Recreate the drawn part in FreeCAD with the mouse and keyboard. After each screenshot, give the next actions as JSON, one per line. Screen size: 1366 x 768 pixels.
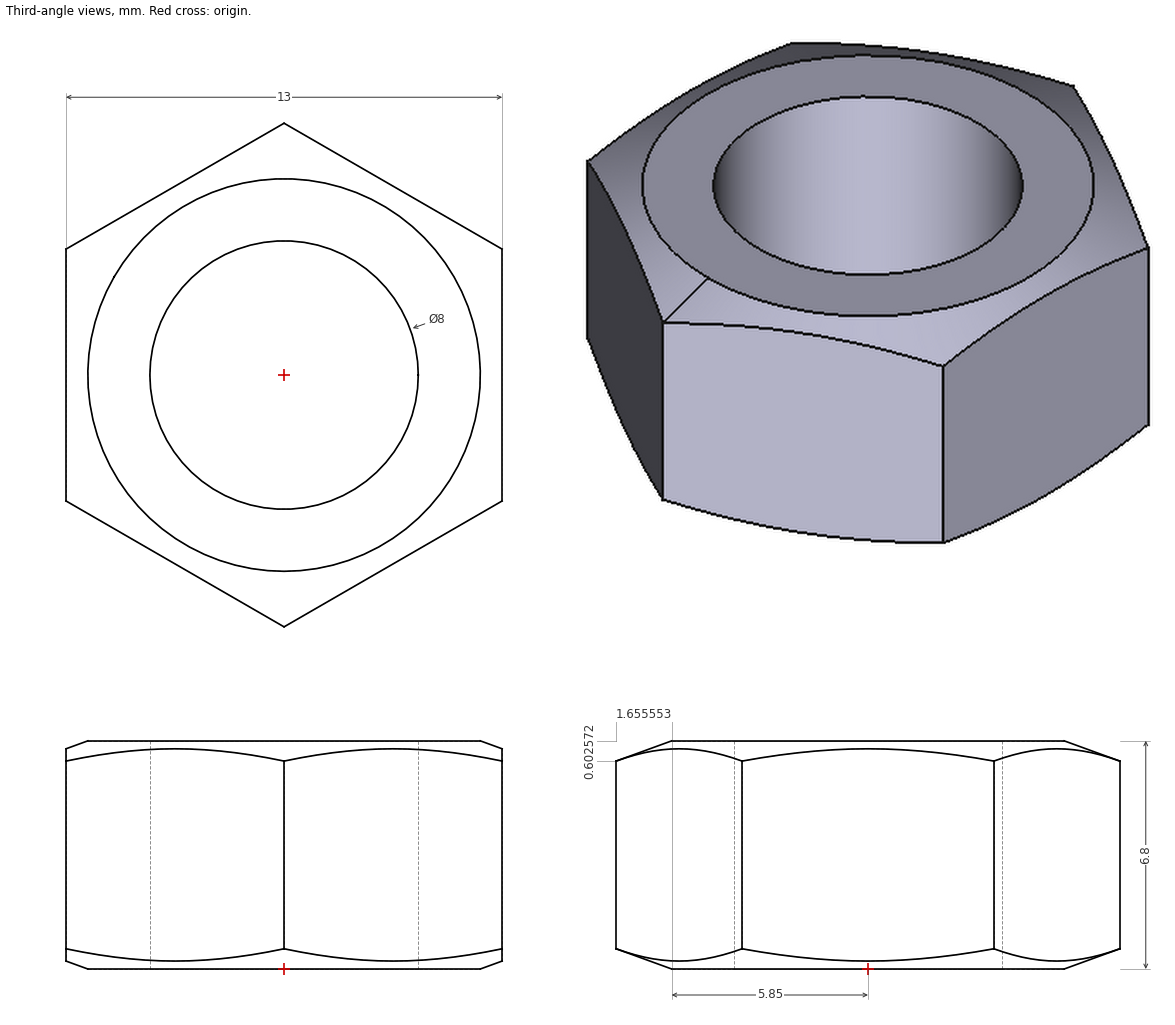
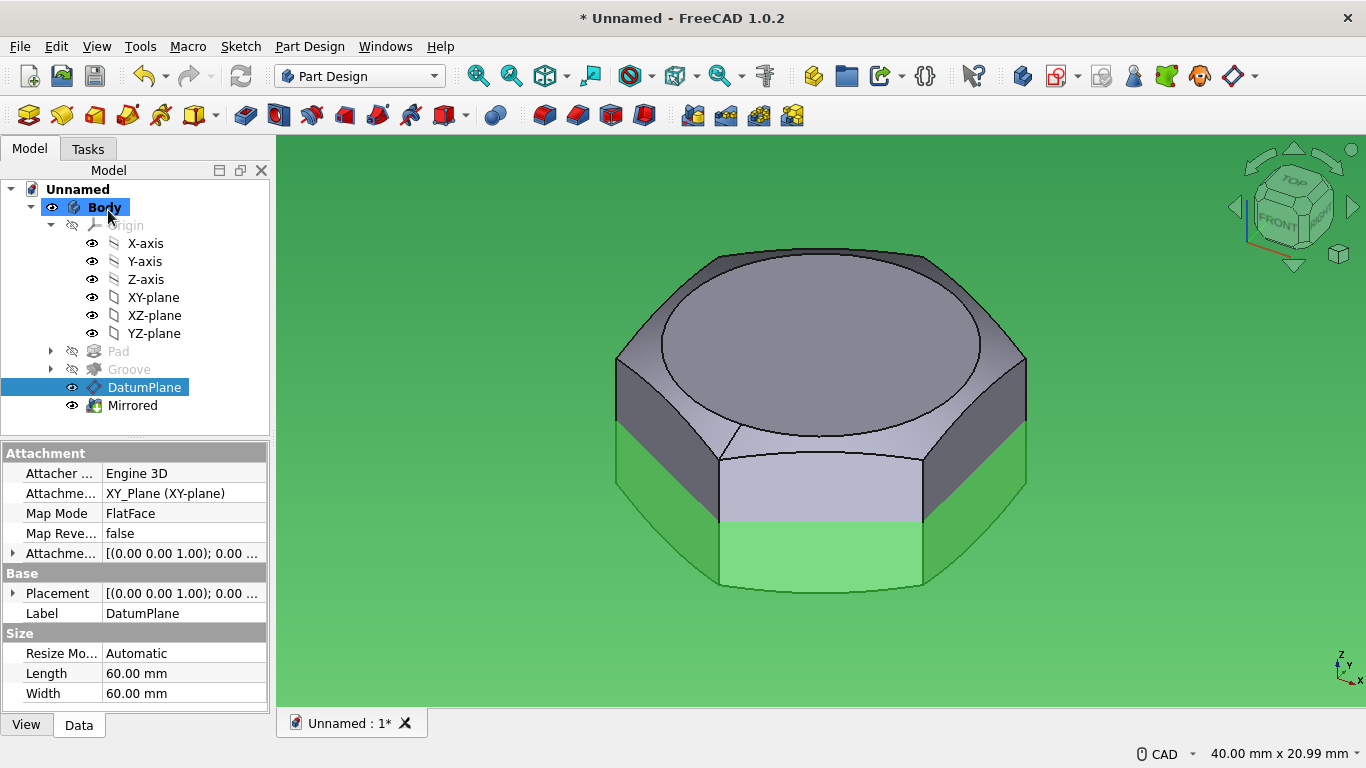
{"action": "left_click", "coordinate": [117, 387]}
{"action": "key", "text": "space"}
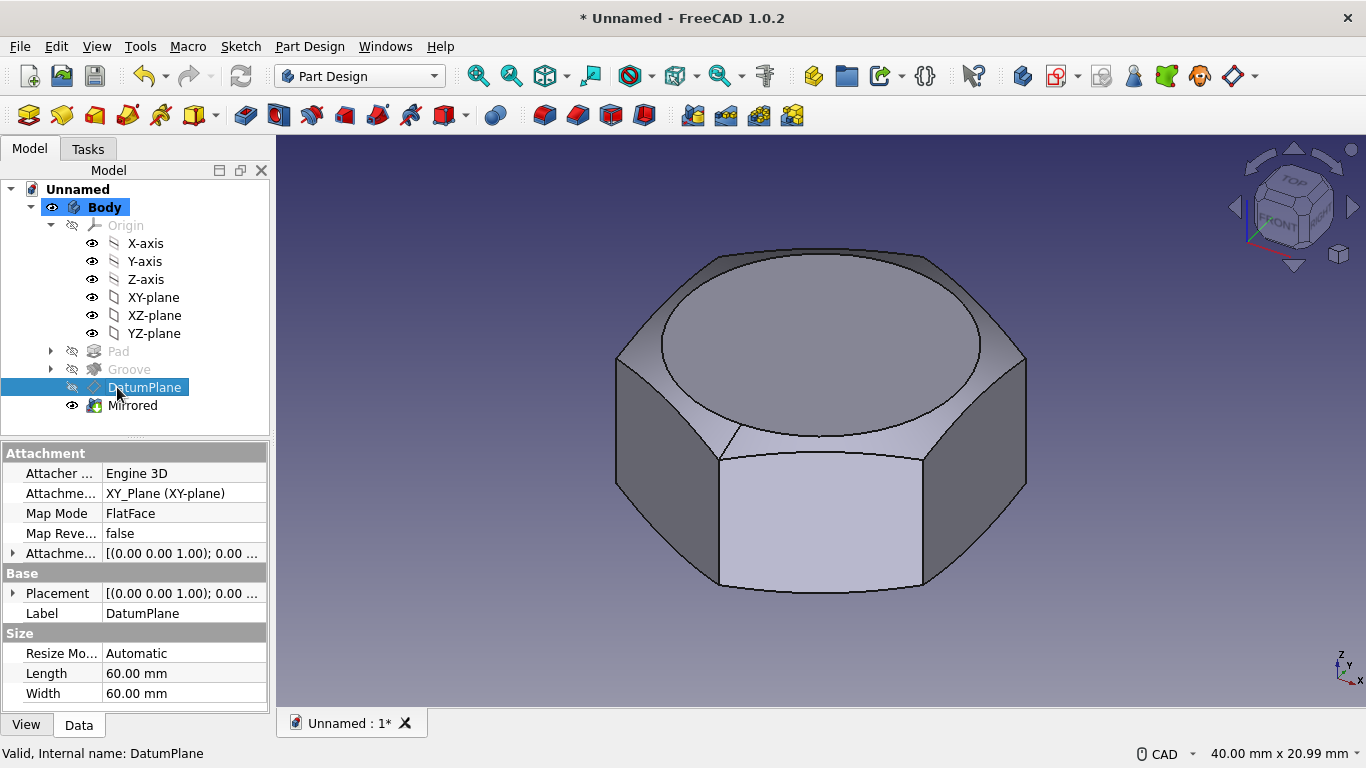
{"action": "left_click", "coordinate": [821, 344]}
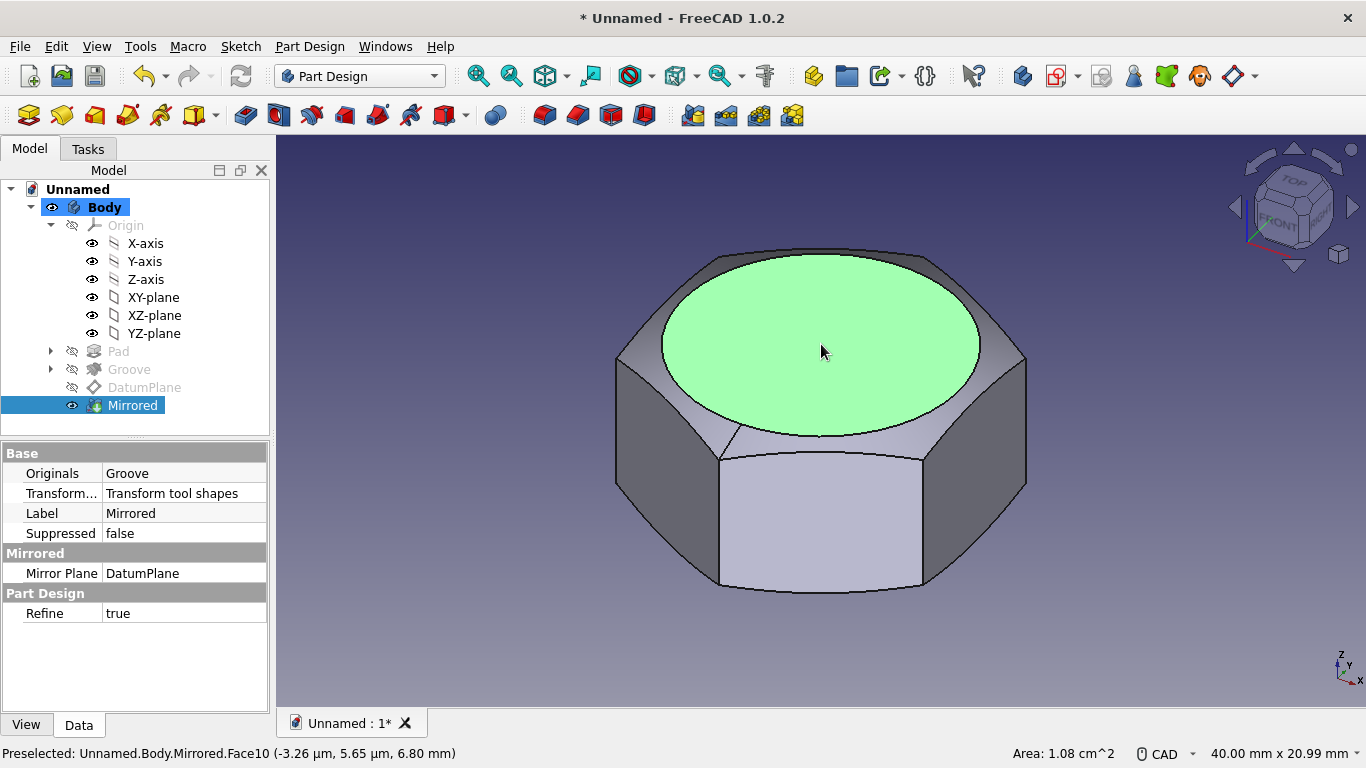
{"action": "left_click", "coordinate": [1056, 76]}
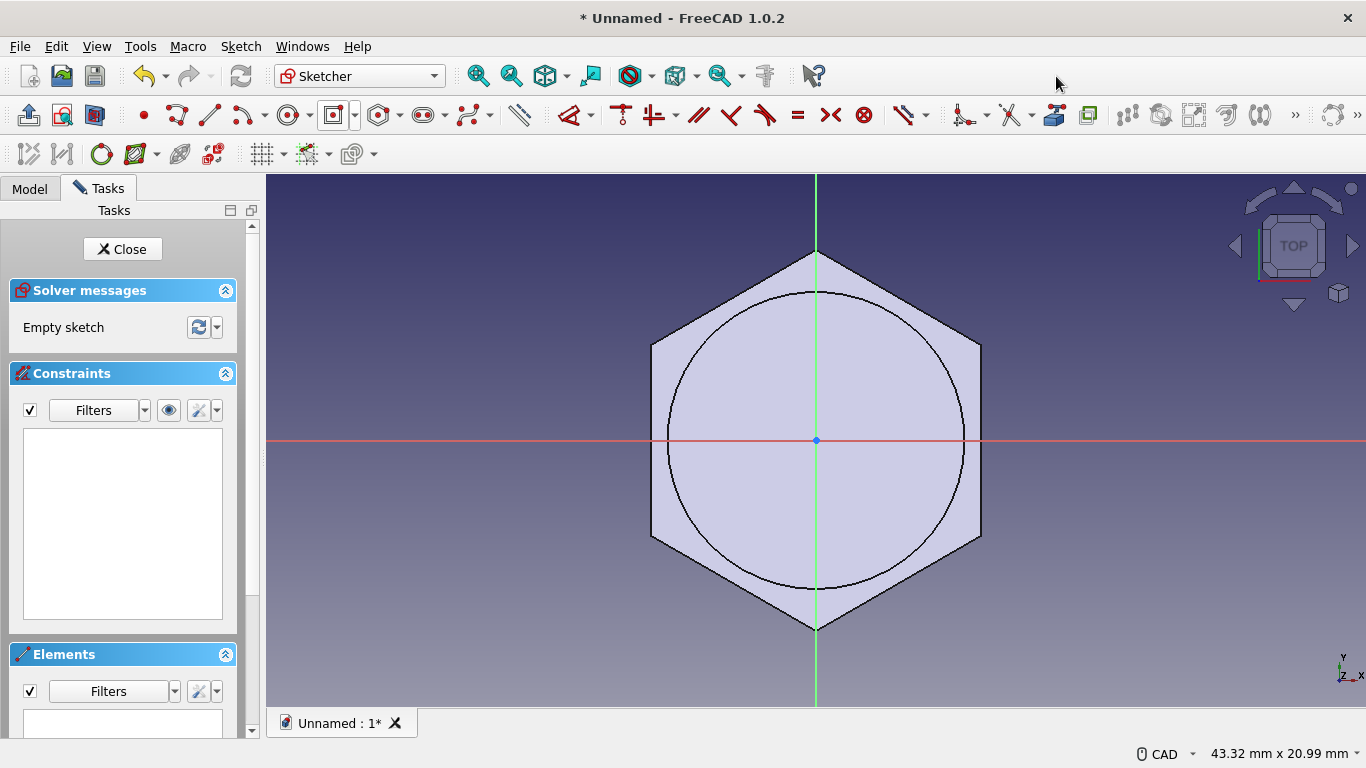
{"action": "scroll", "coordinate": [899, 441], "scroll_direction": "up", "scroll_amount": 3}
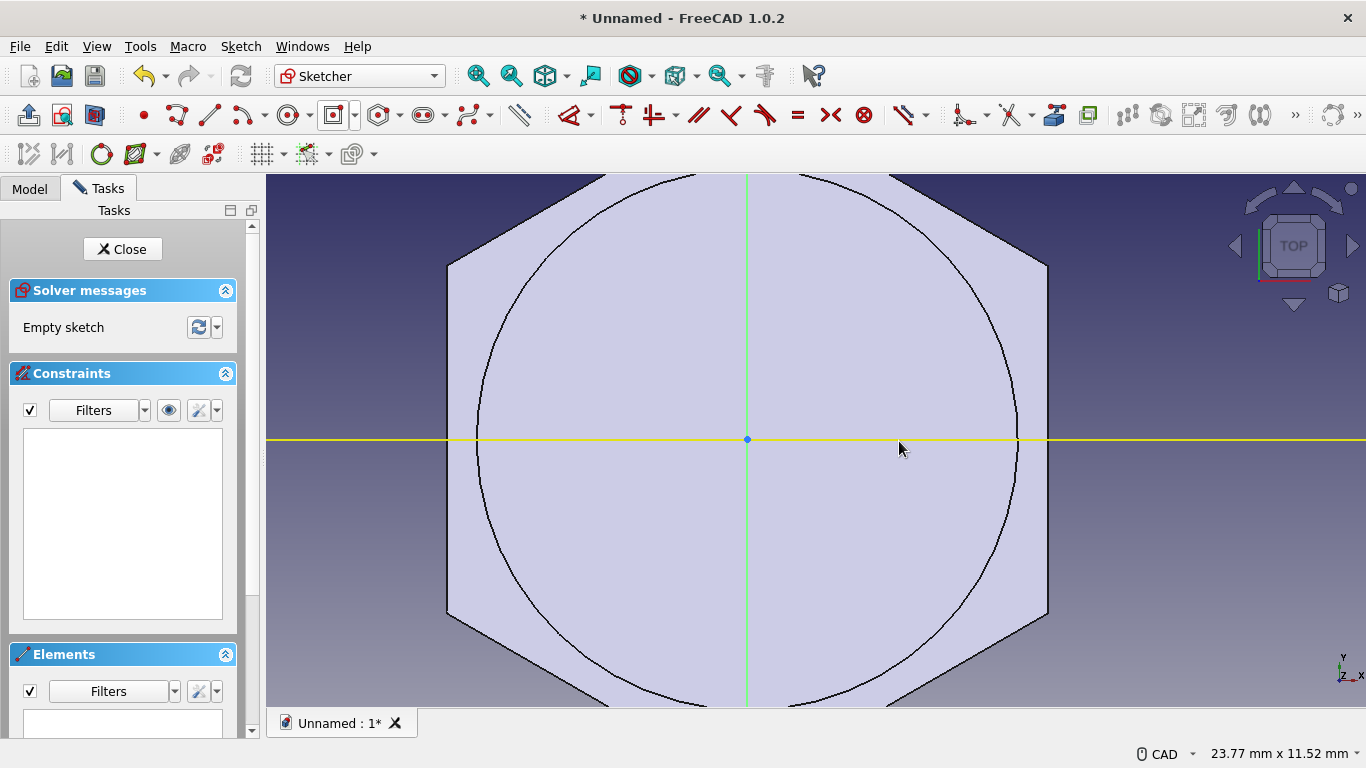
{"action": "left_click", "coordinate": [288, 116]}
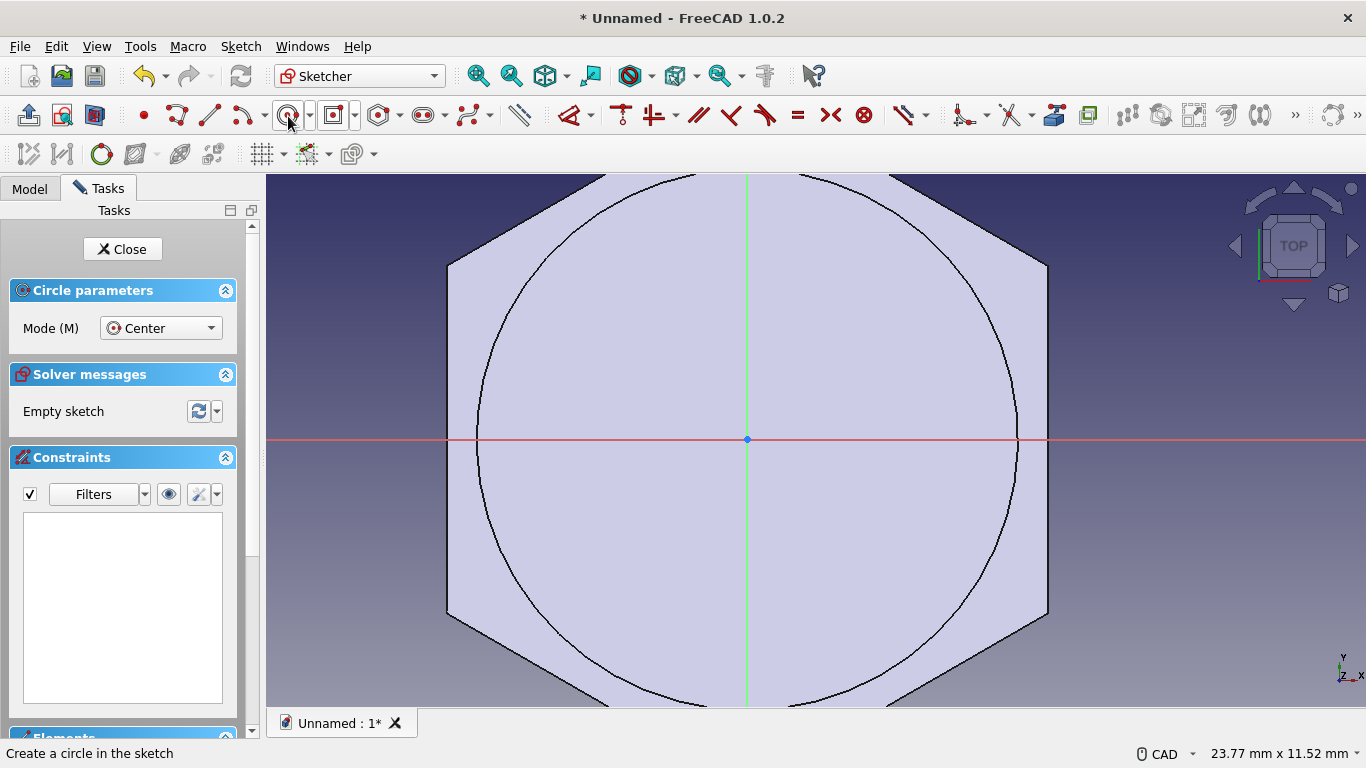
{"action": "left_click", "coordinate": [747, 440]}
{"action": "left_click", "coordinate": [878, 309]}
{"action": "key", "text": "Escape"}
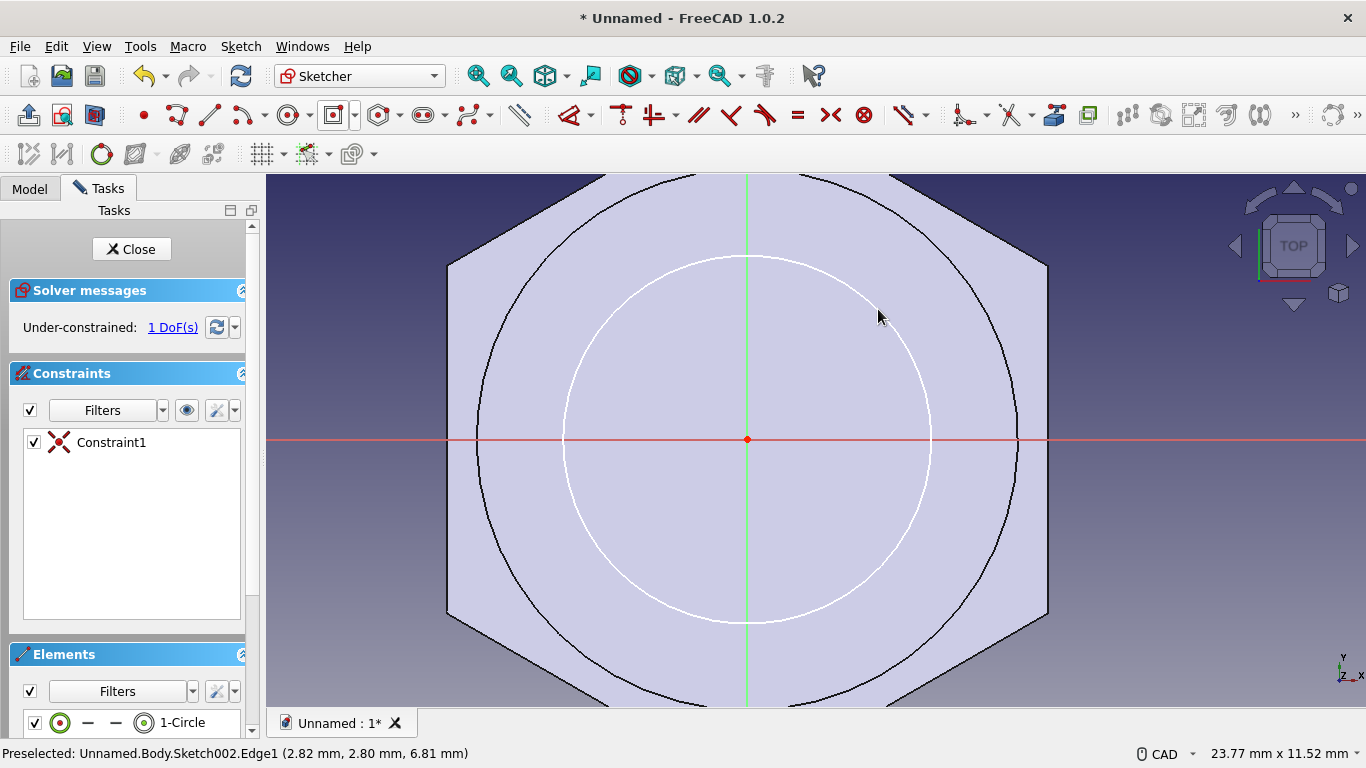
{"action": "key", "text": "d"}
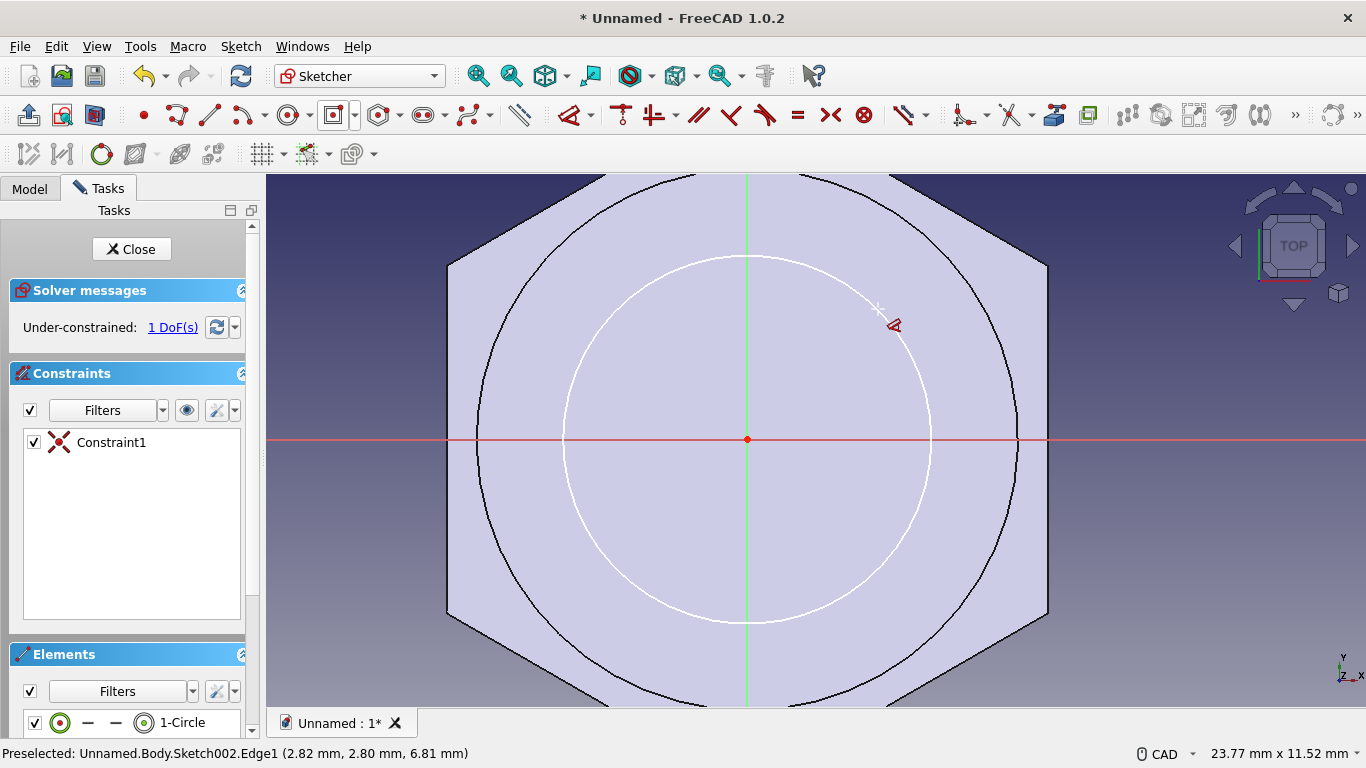
{"action": "left_click", "coordinate": [877, 309]}
{"action": "left_click", "coordinate": [900, 286]}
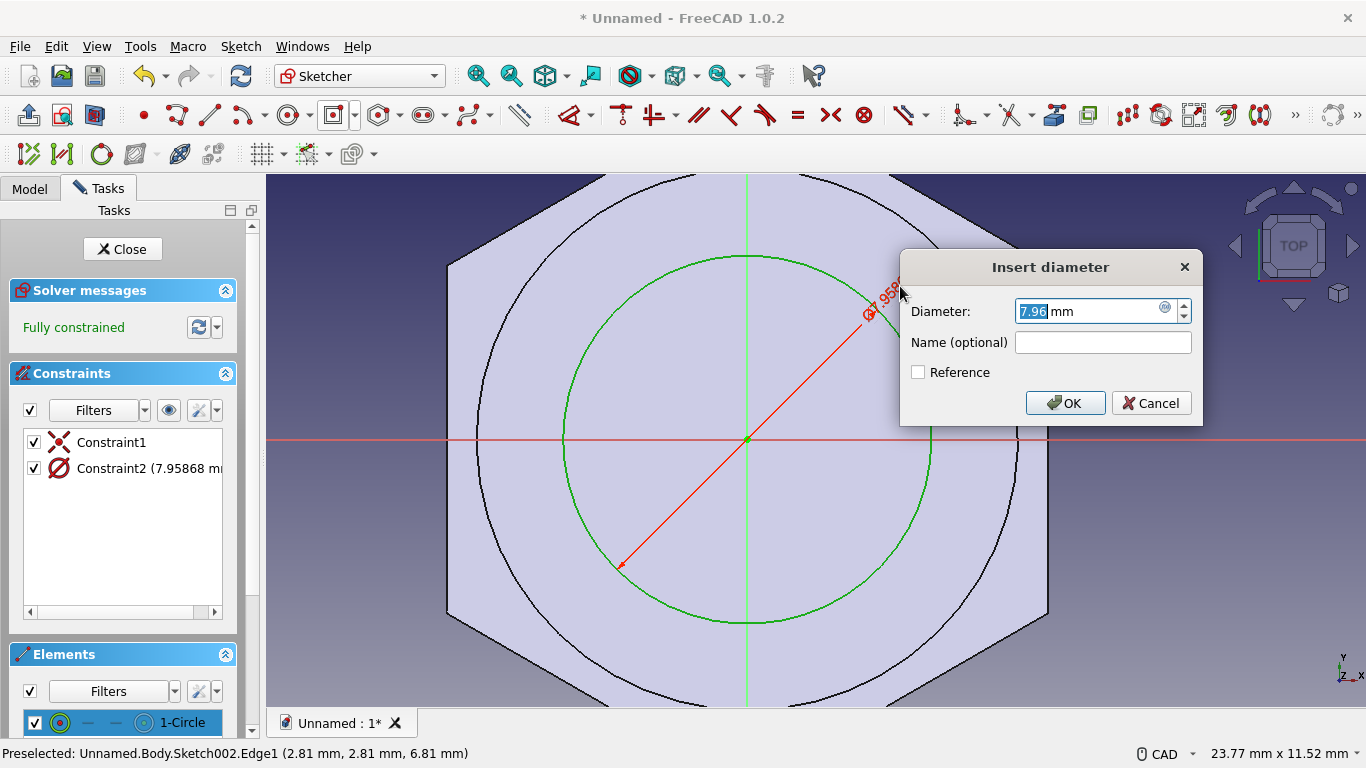
{"action": "type", "text": "8"}
{"action": "key", "text": "Return"}
{"action": "key", "text": "Escape"}